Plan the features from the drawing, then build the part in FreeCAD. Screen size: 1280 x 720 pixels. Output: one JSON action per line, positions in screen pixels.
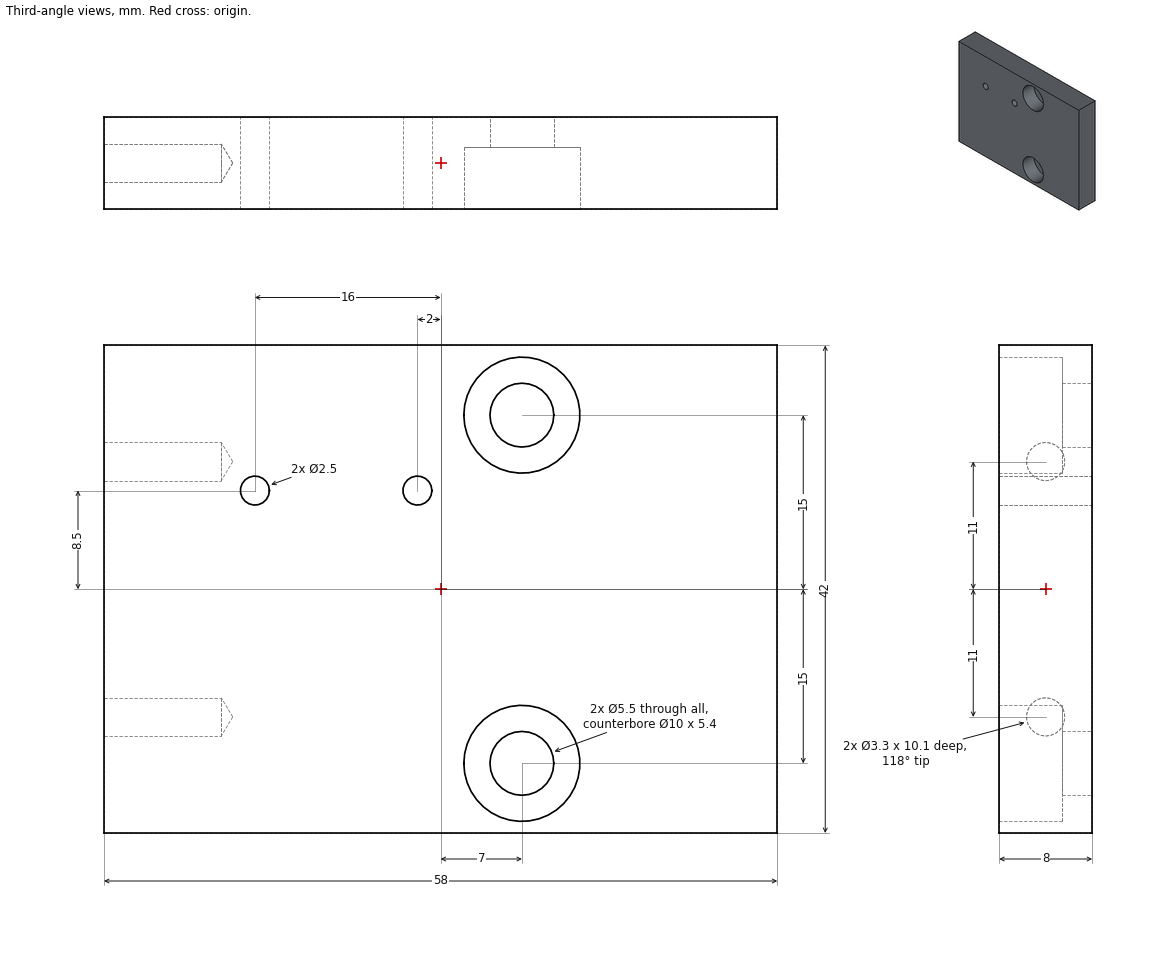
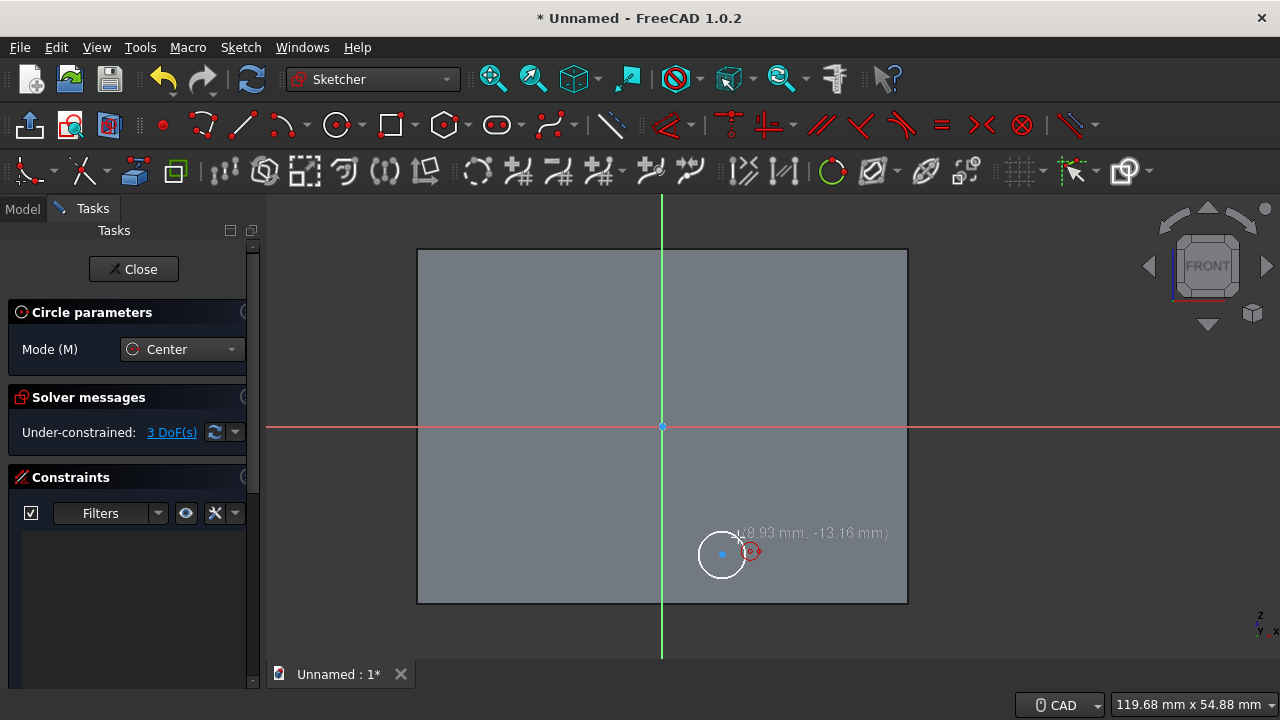
{"action": "left_click", "coordinate": [722, 299]}
{"action": "left_click", "coordinate": [738, 283]}
{"action": "key", "text": "Escape"}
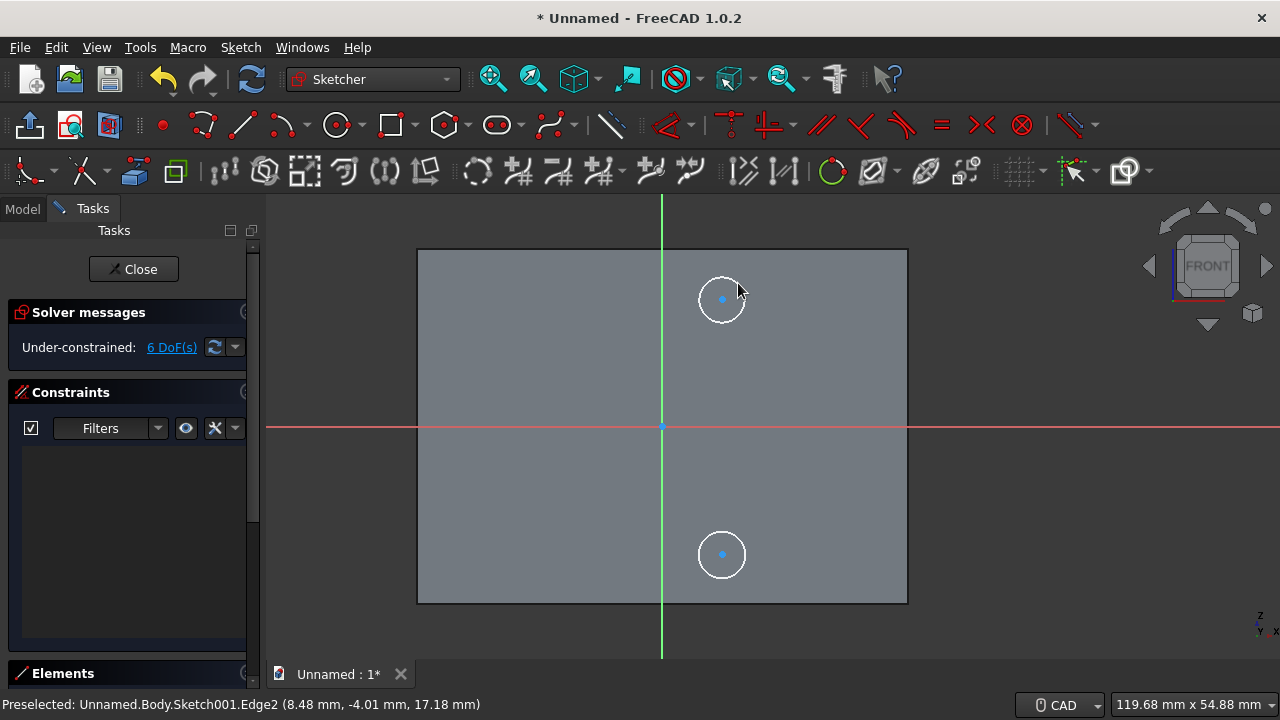
{"action": "left_click", "coordinate": [738, 538]}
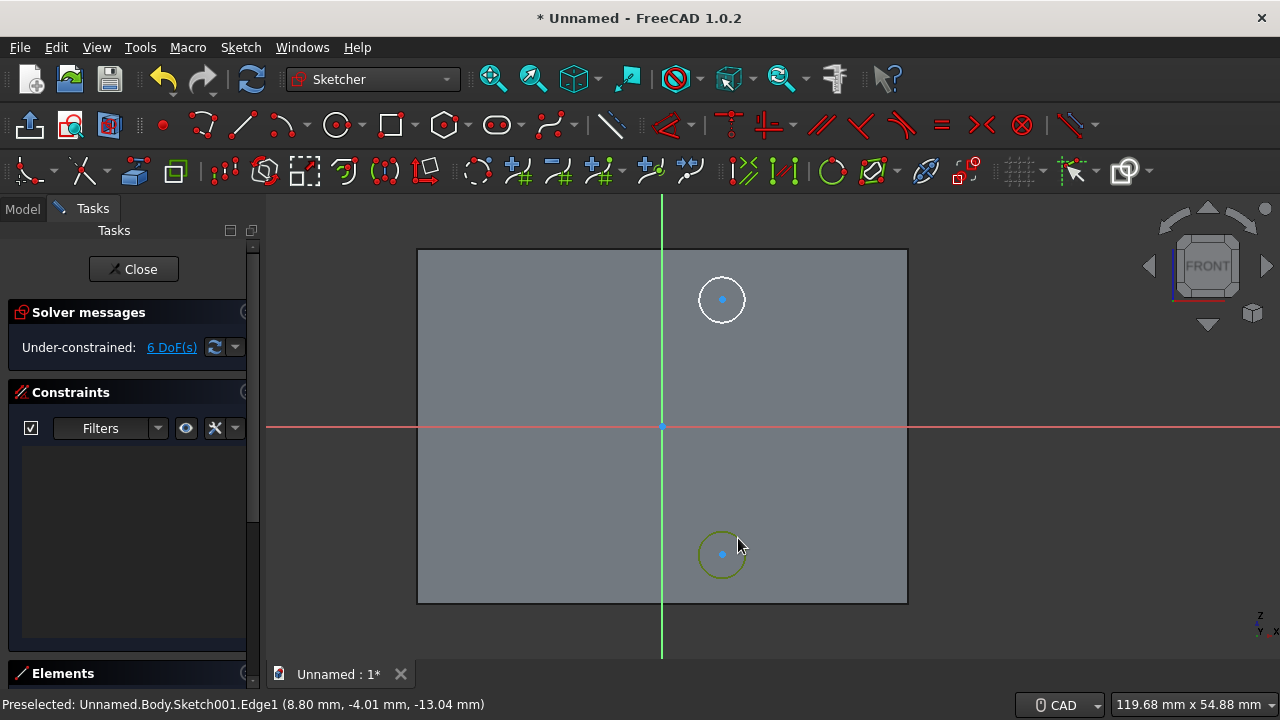
{"action": "left_click", "coordinate": [738, 284]}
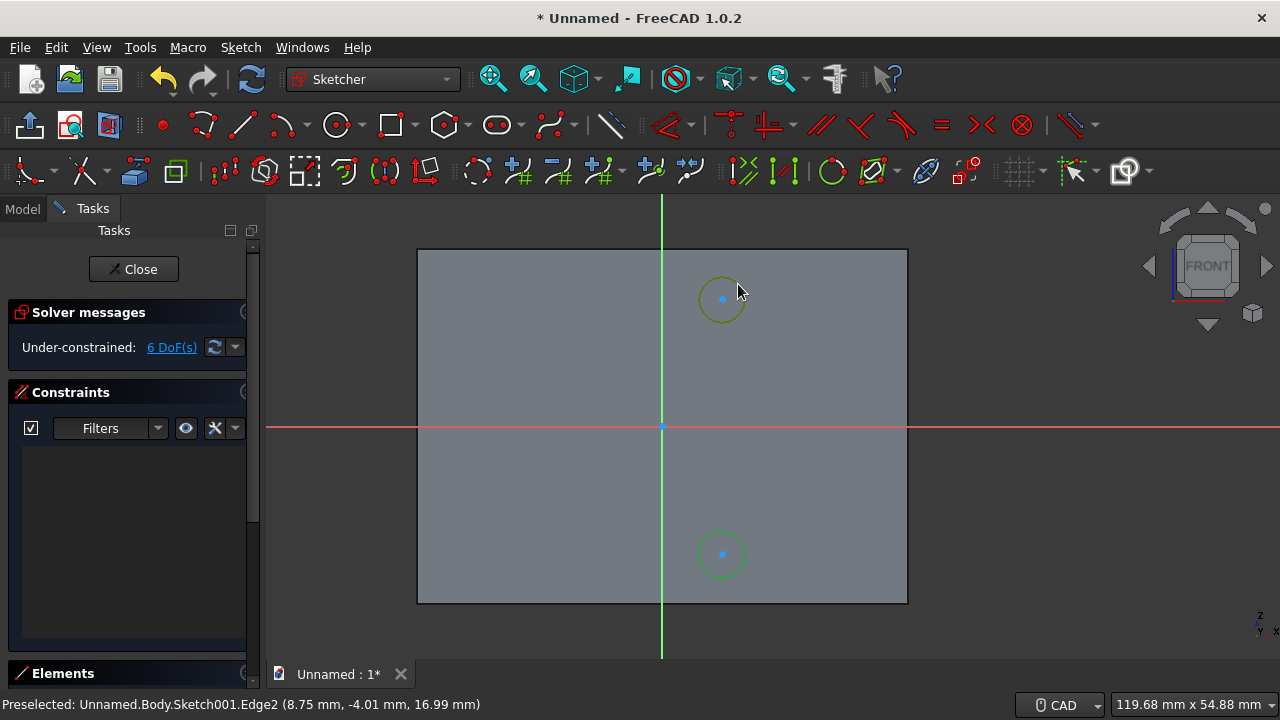
{"action": "left_click", "coordinate": [942, 126]}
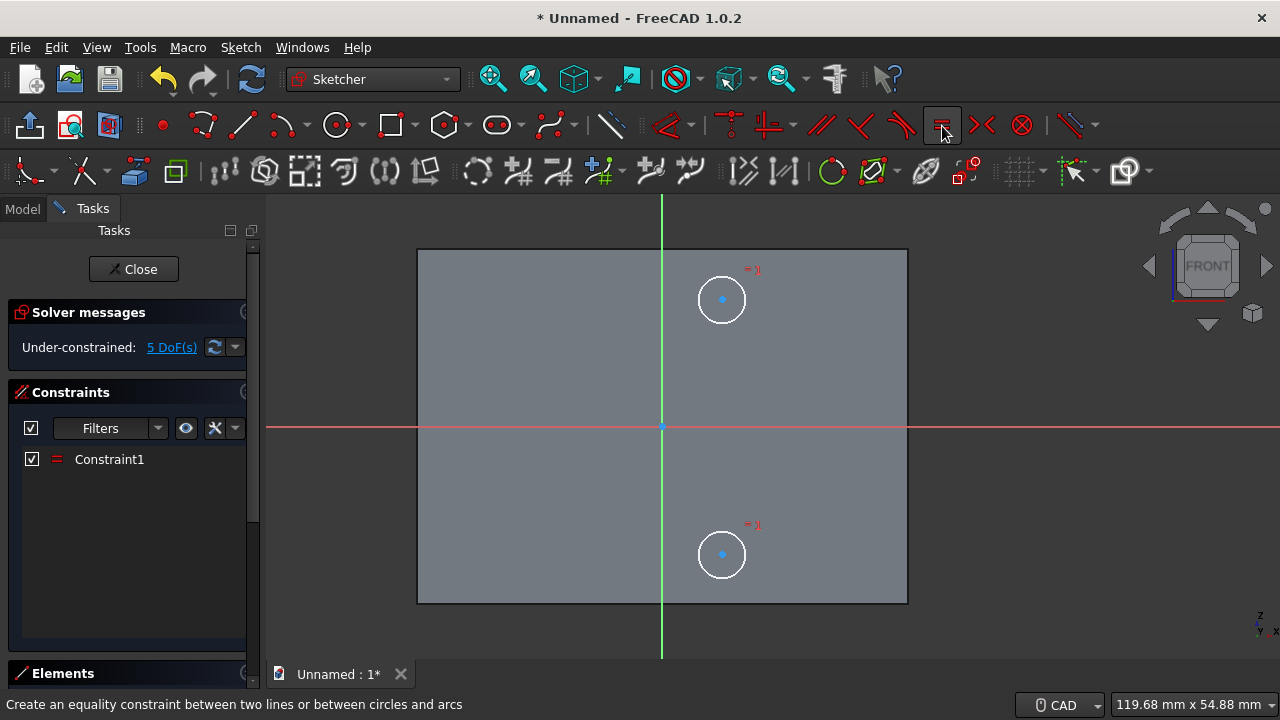
{"action": "left_click", "coordinate": [722, 555]}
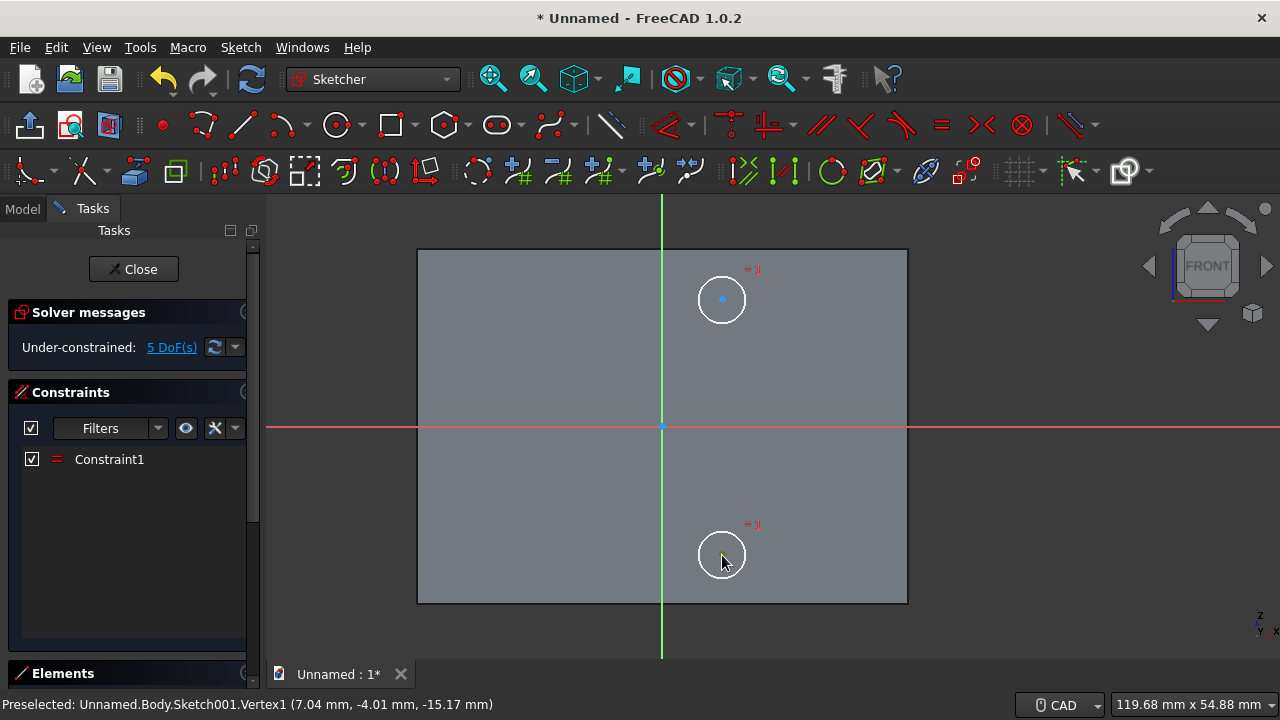
{"action": "left_click", "coordinate": [722, 300]}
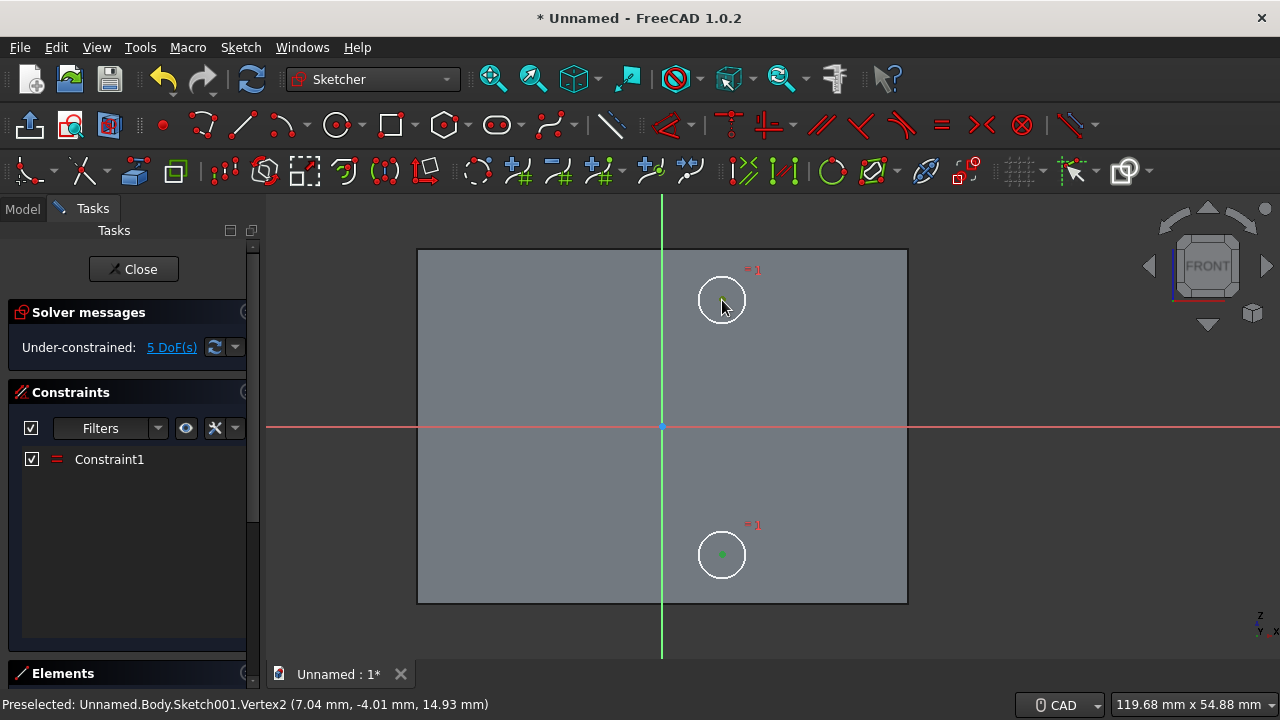
{"action": "key", "text": "v"}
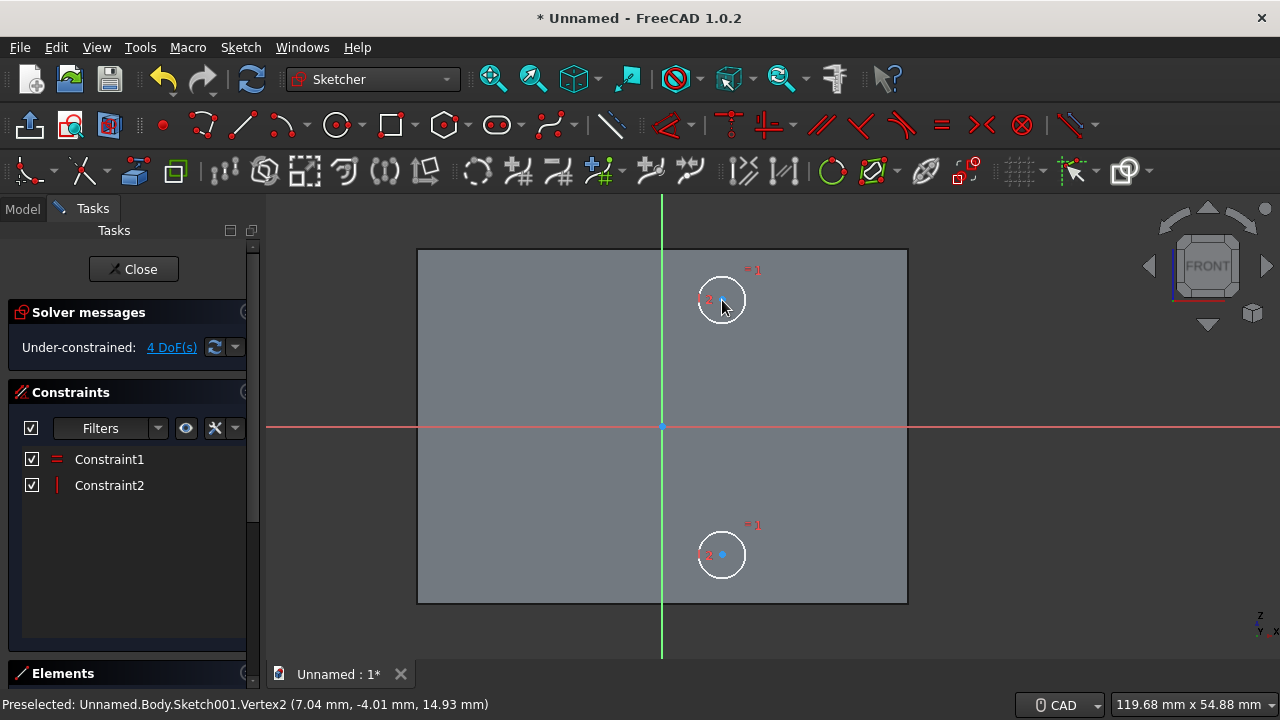
{"action": "left_click", "coordinate": [666, 126]}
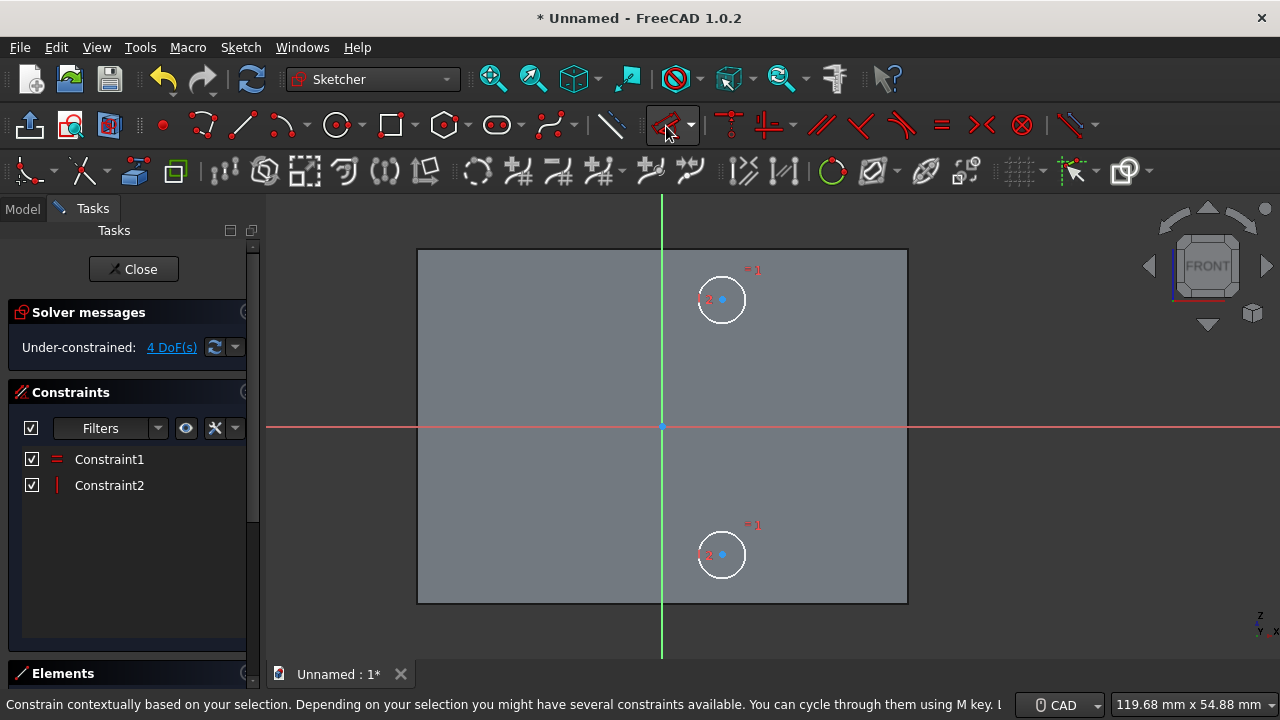
{"action": "left_click", "coordinate": [738, 538]}
{"action": "left_click", "coordinate": [760, 515]}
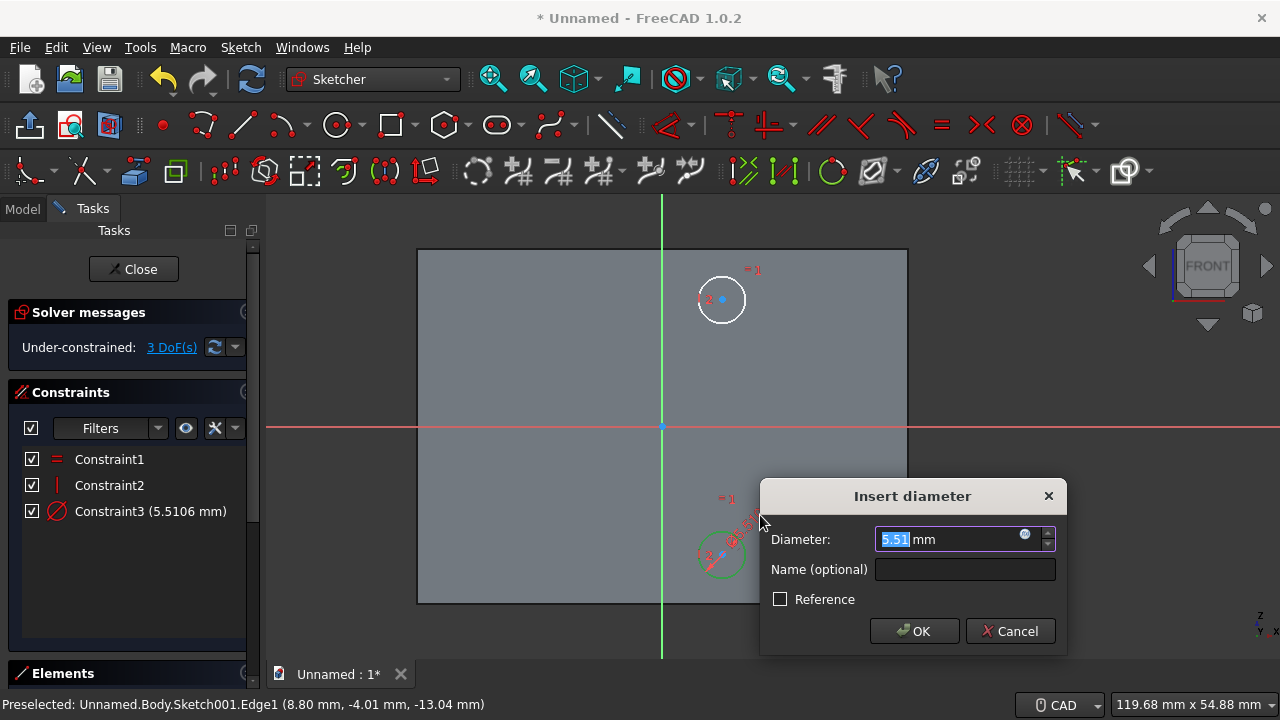
{"action": "type", "text": "5.5"}
{"action": "key", "text": "Return"}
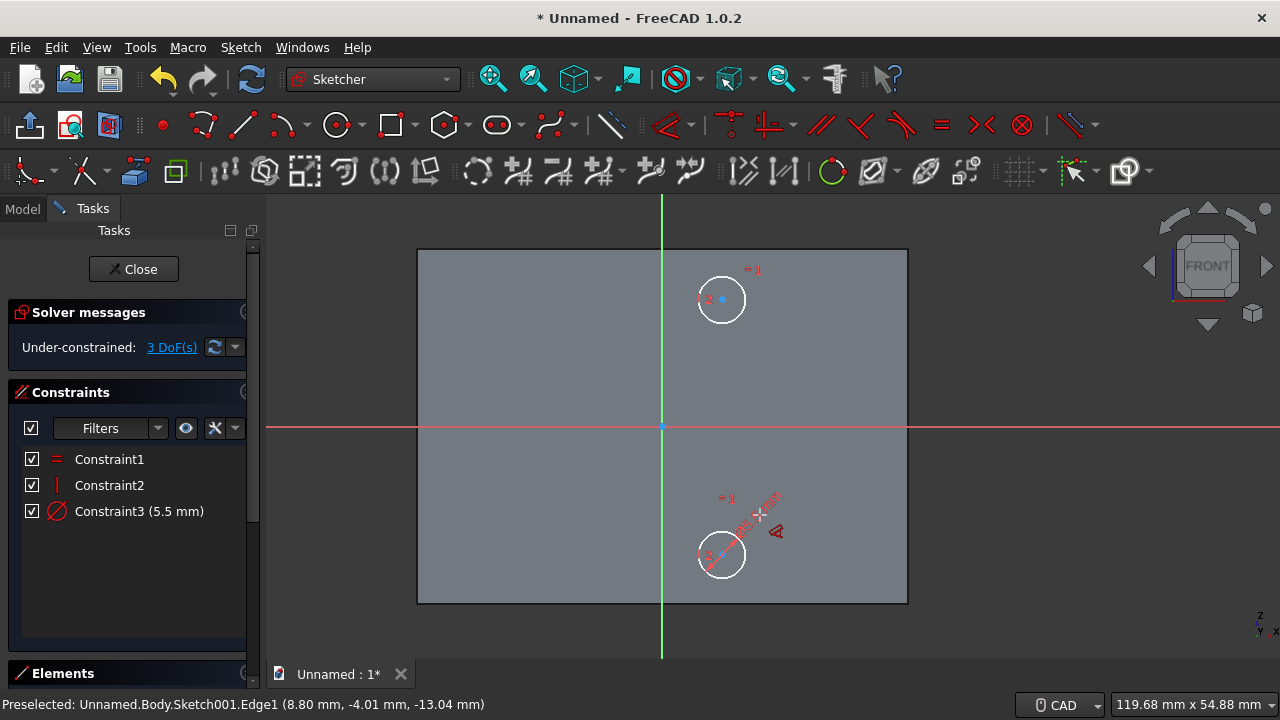
{"action": "left_click", "coordinate": [722, 555]}
{"action": "left_click", "coordinate": [692, 589]}